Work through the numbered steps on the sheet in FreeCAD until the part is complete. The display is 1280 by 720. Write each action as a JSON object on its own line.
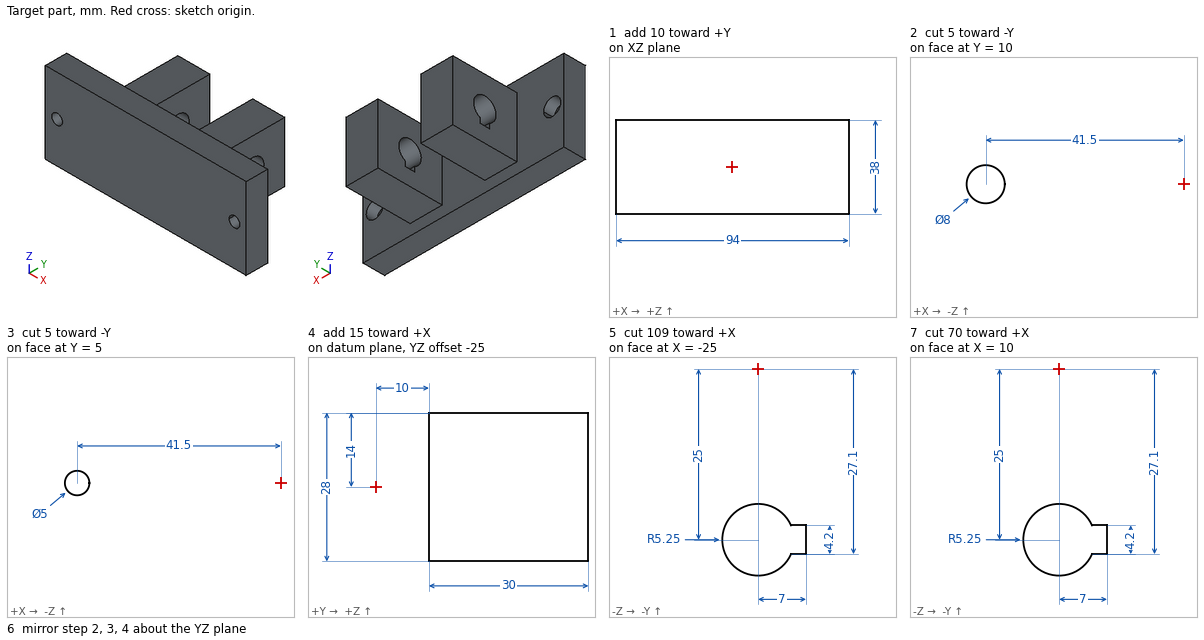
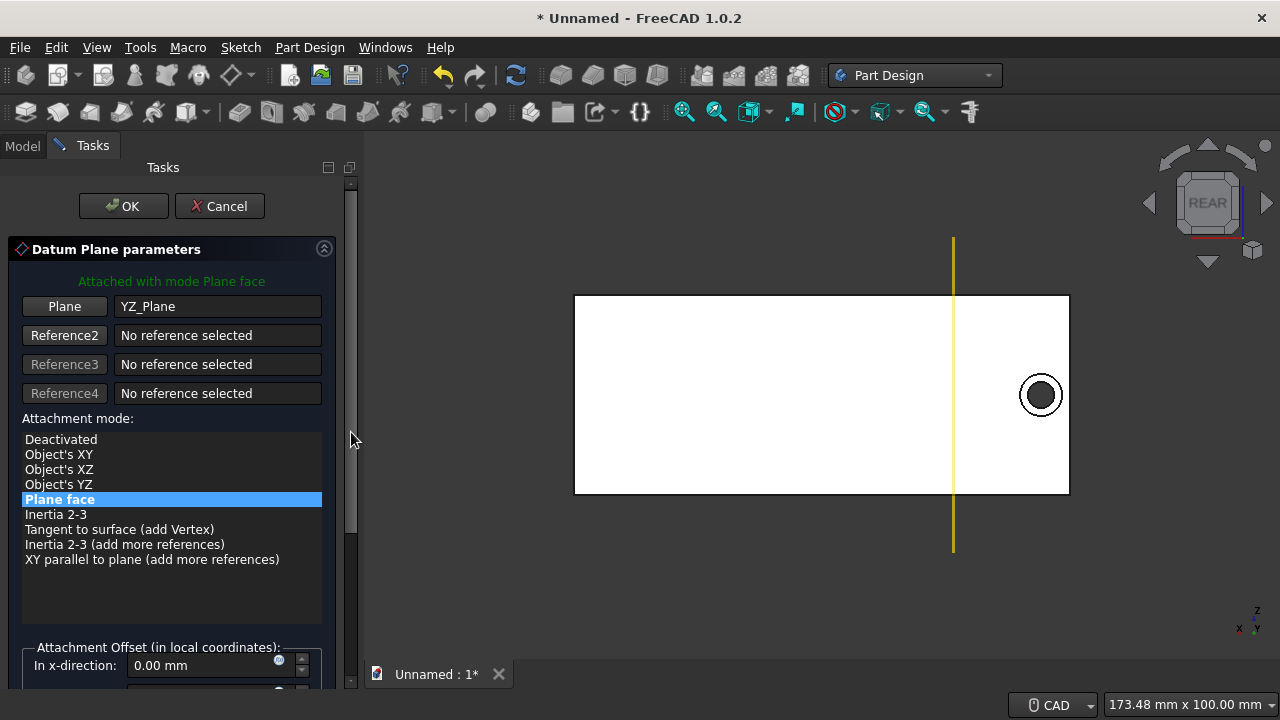
{"action": "left_click", "coordinate": [124, 206]}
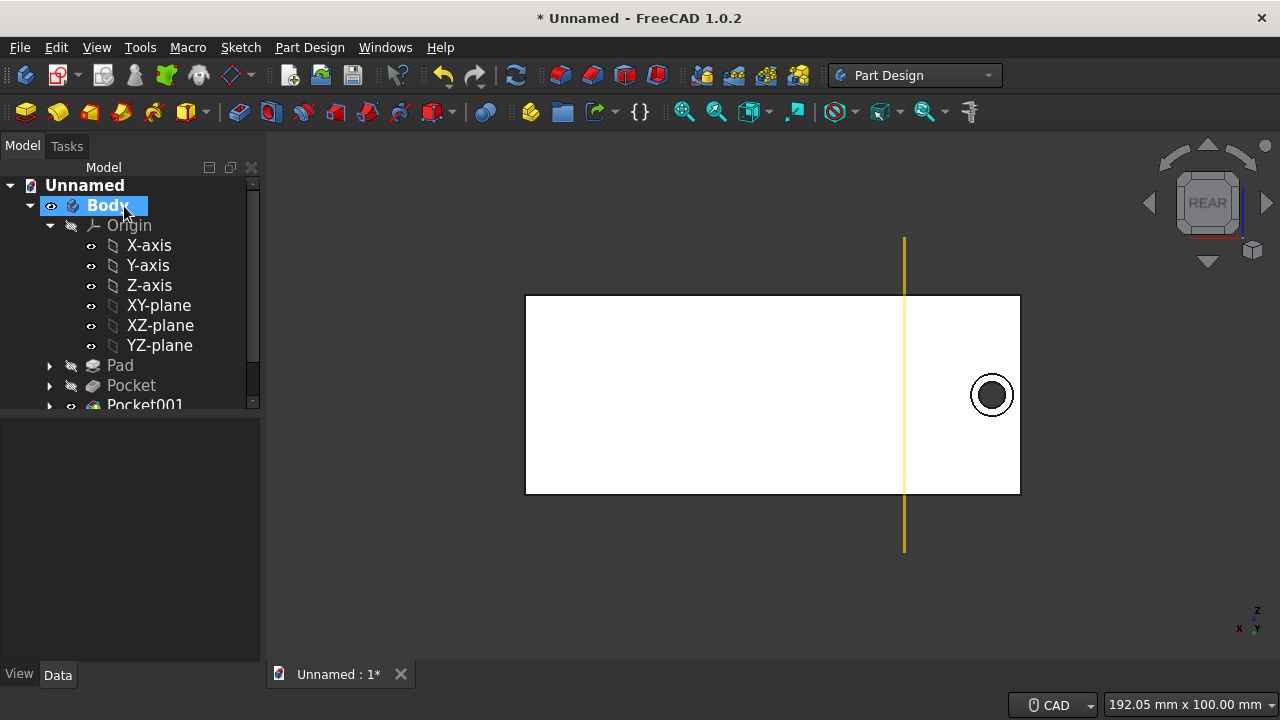
{"action": "scroll", "coordinate": [100, 301], "scroll_direction": "down", "scroll_amount": 3}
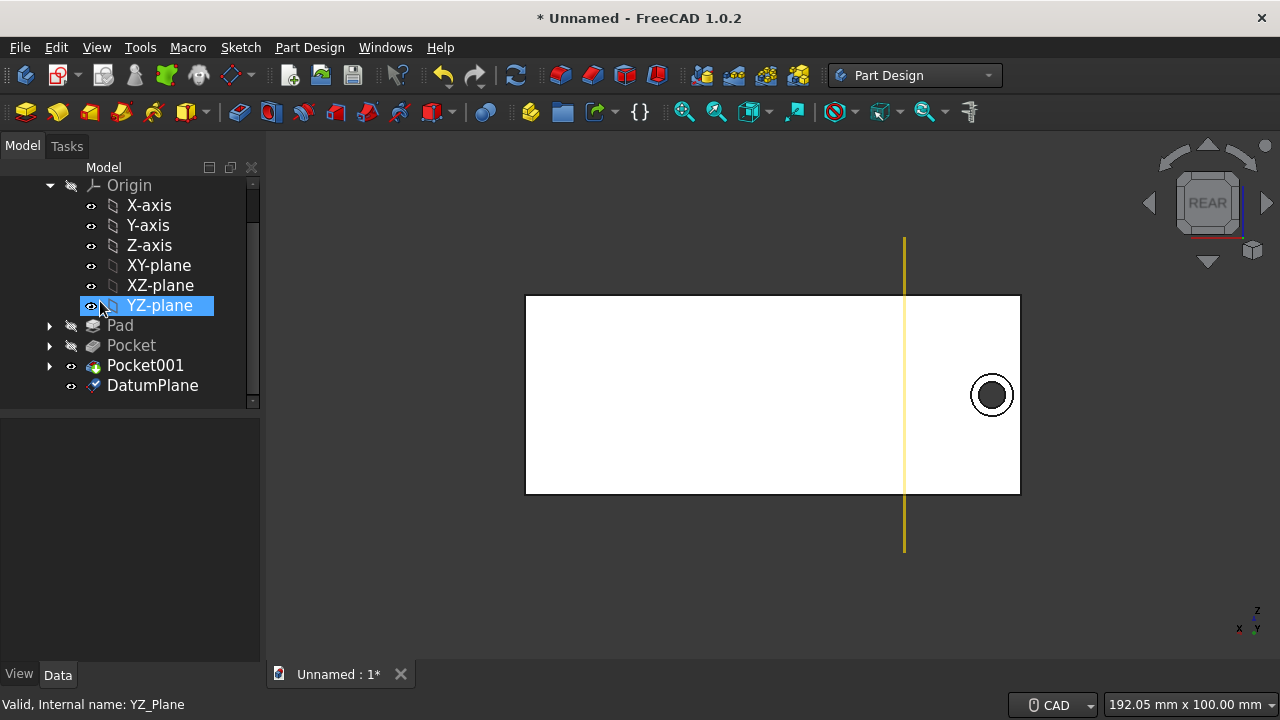
{"action": "left_click", "coordinate": [116, 386]}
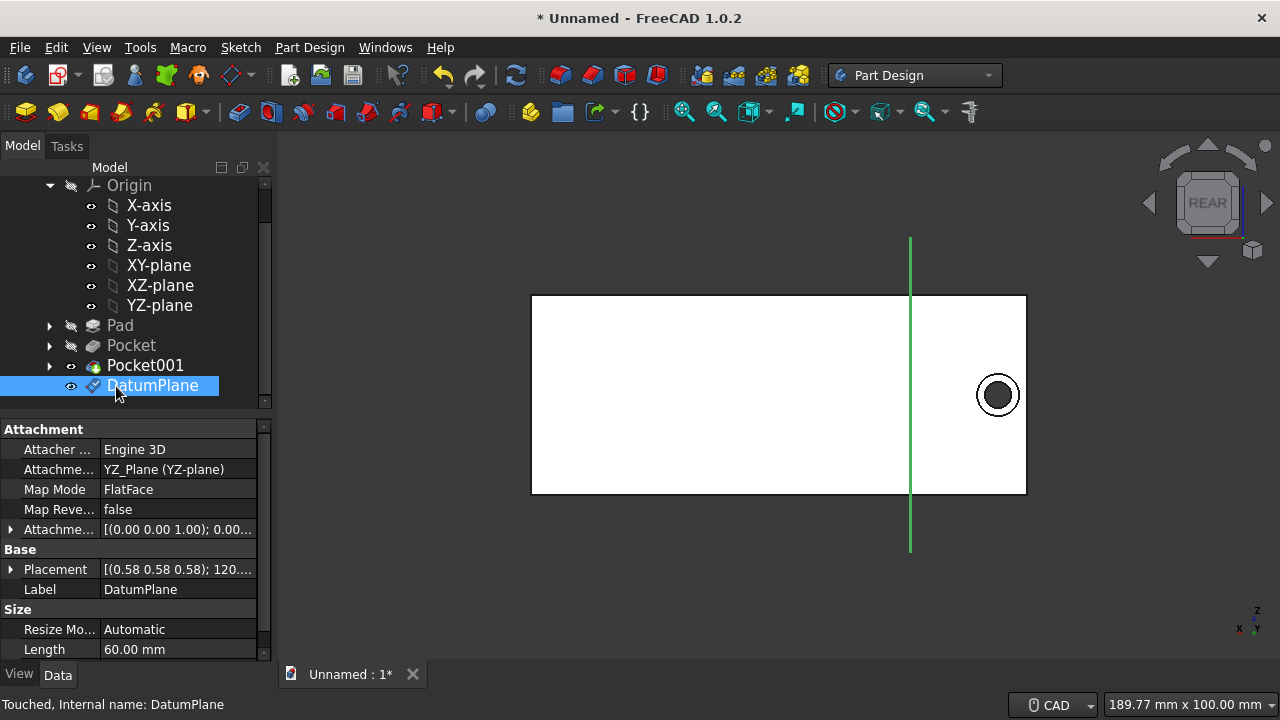
{"action": "left_click", "coordinate": [58, 76]}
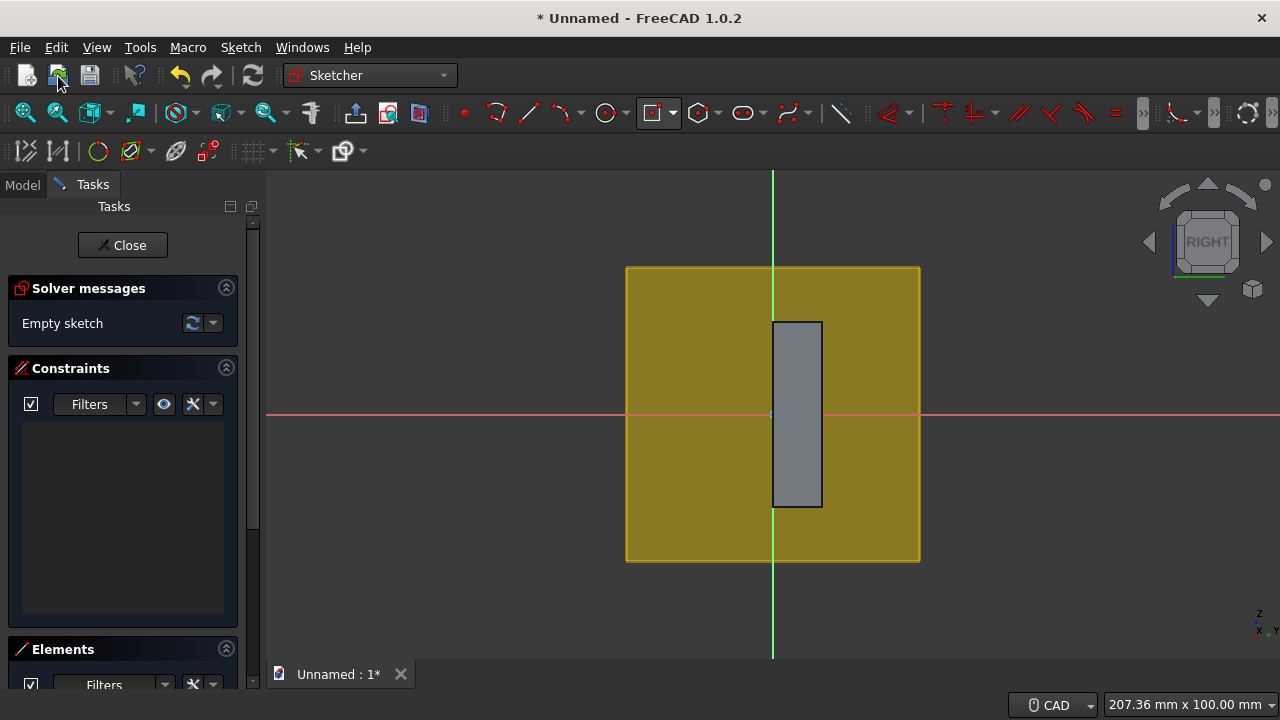
{"action": "left_click", "coordinate": [420, 114]}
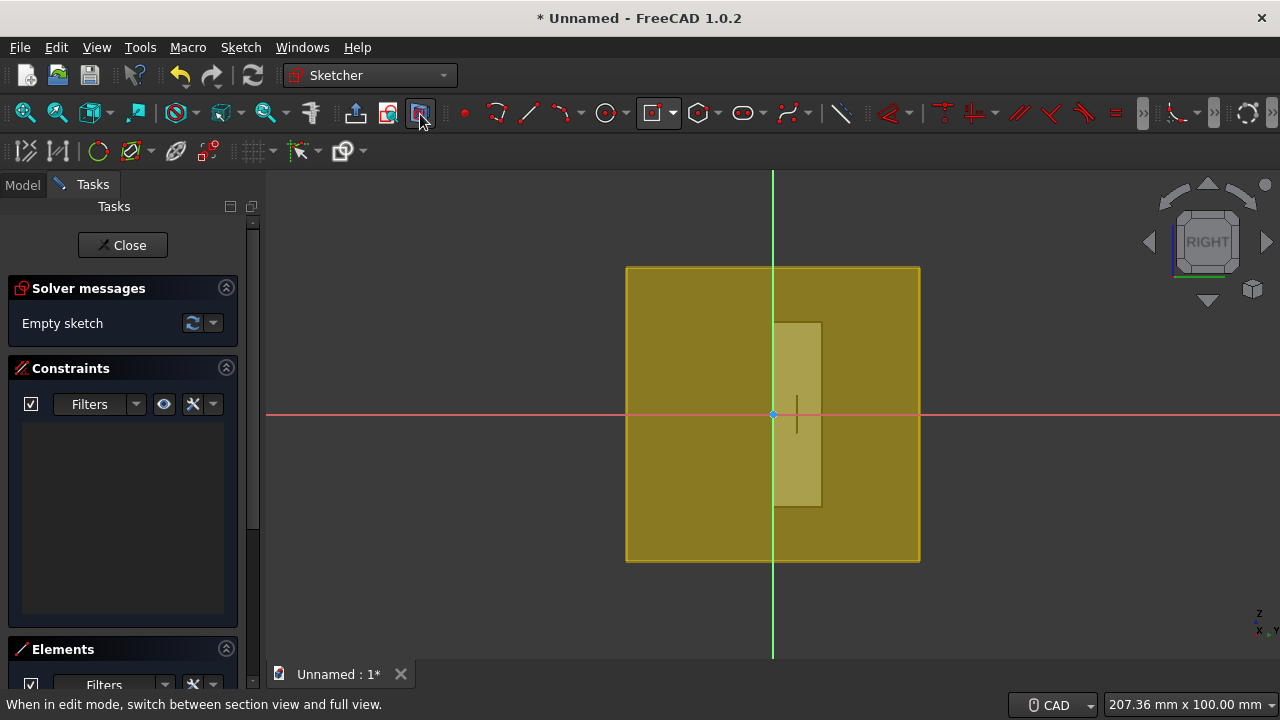
{"action": "scroll", "coordinate": [1006, 415], "scroll_direction": "up", "scroll_amount": 4}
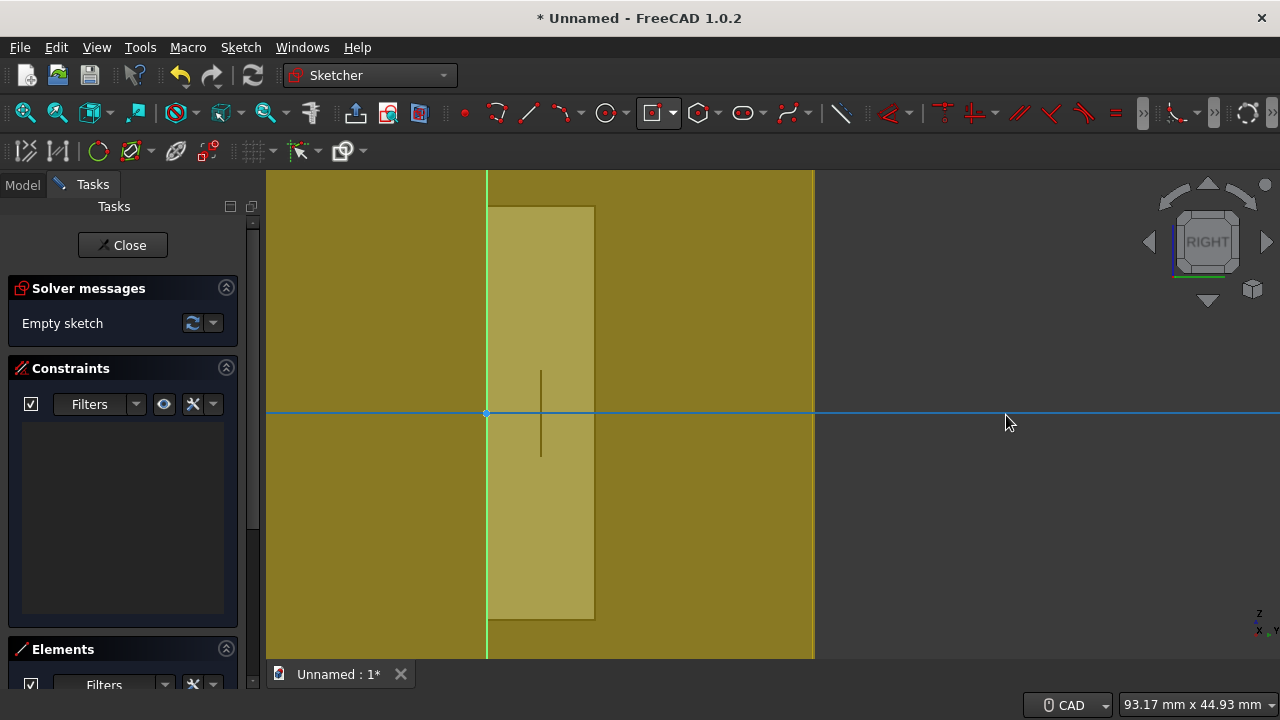
{"action": "left_click", "coordinate": [676, 114]}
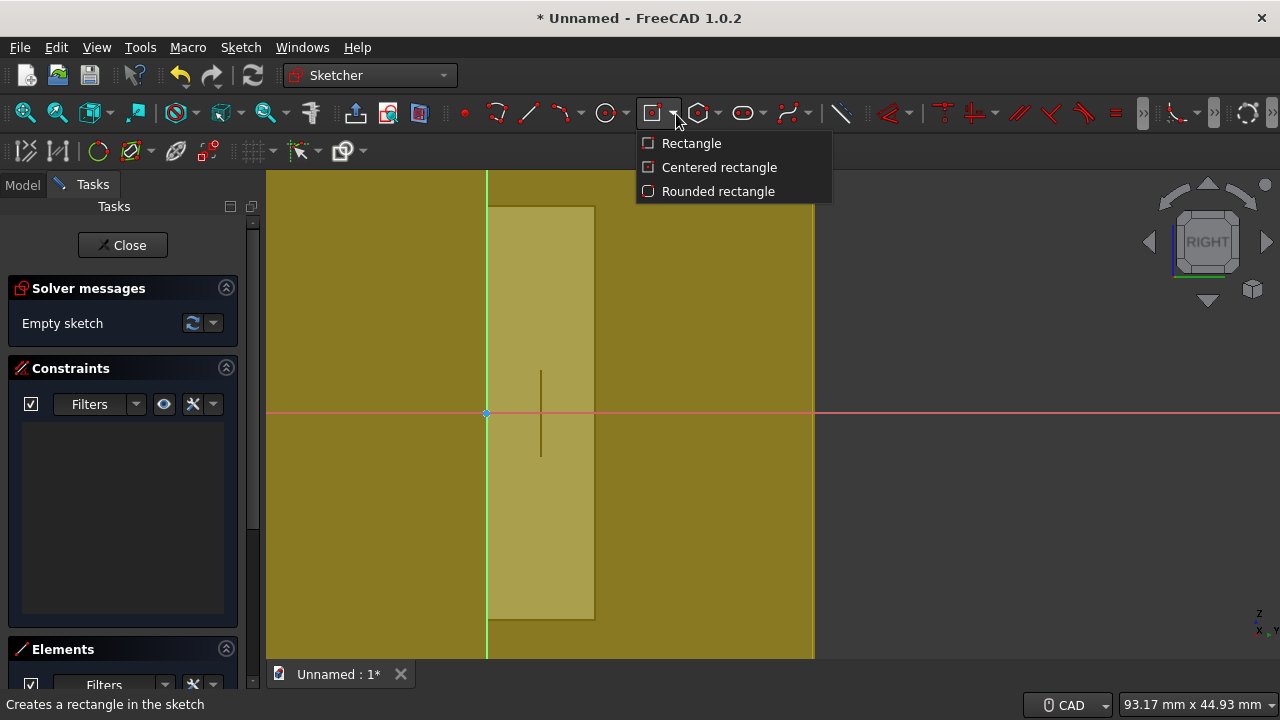
{"action": "left_click", "coordinate": [734, 143]}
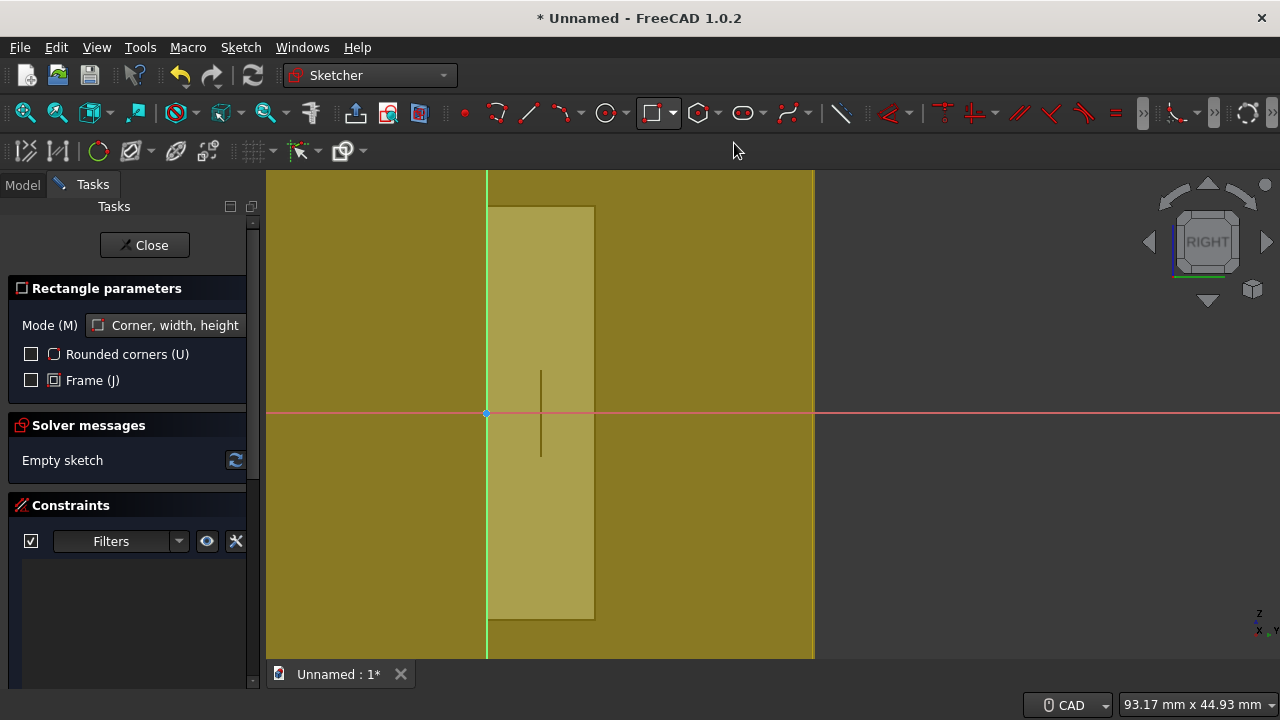
{"action": "left_click", "coordinate": [595, 261]}
{"action": "left_click", "coordinate": [922, 566]}
{"action": "key", "text": "Escape"}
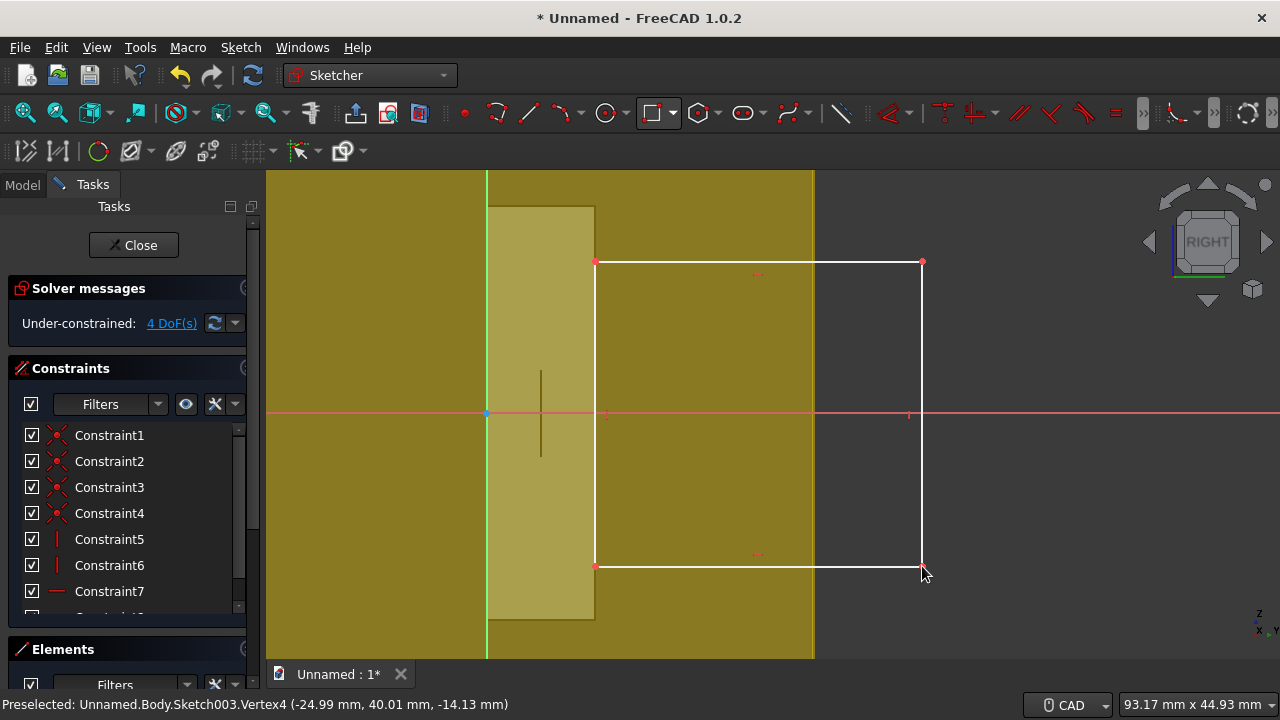
{"action": "left_click", "coordinate": [888, 114]}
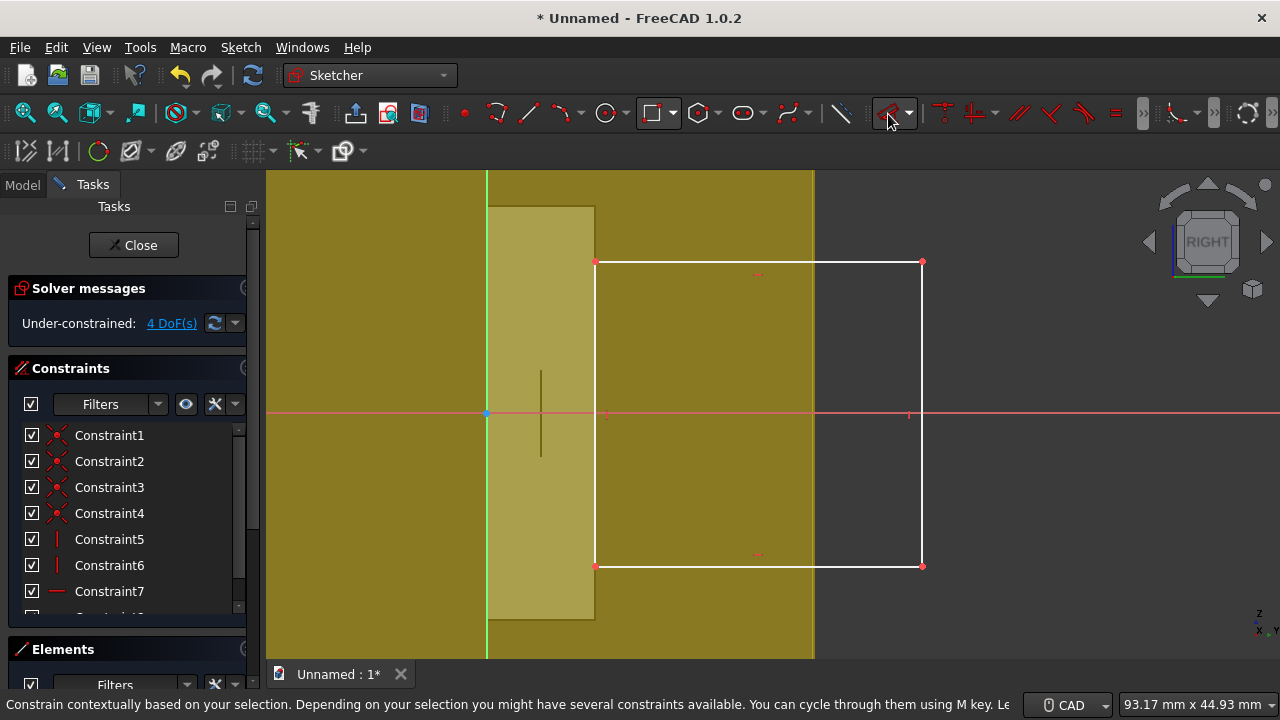
{"action": "left_click", "coordinate": [595, 354]}
{"action": "left_click", "coordinate": [561, 344]}